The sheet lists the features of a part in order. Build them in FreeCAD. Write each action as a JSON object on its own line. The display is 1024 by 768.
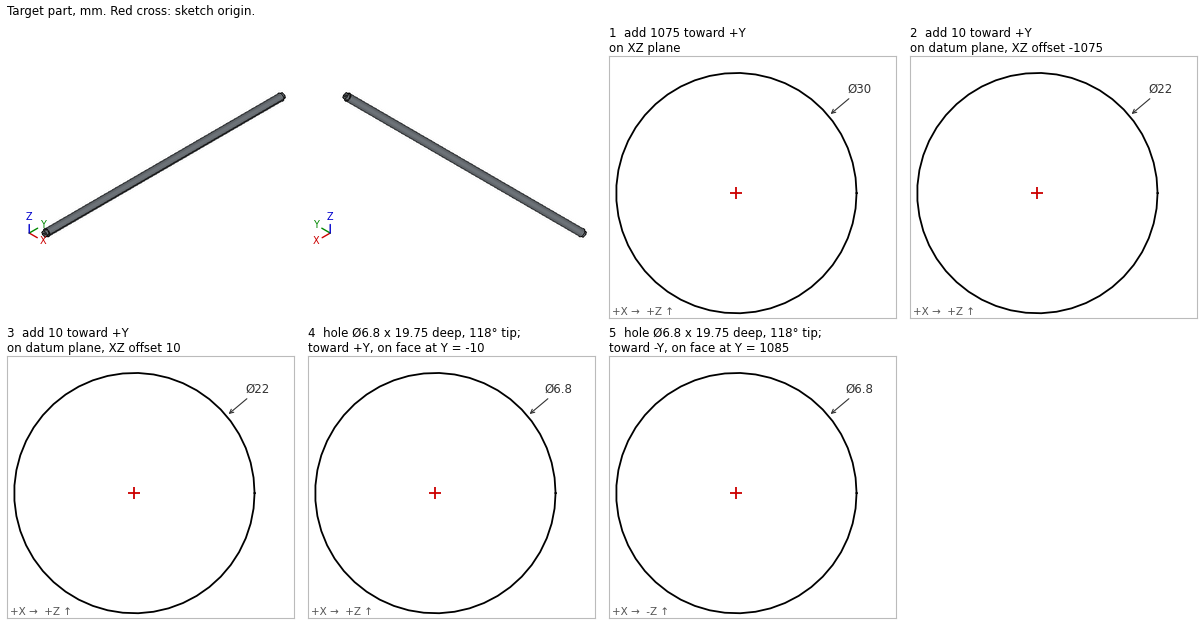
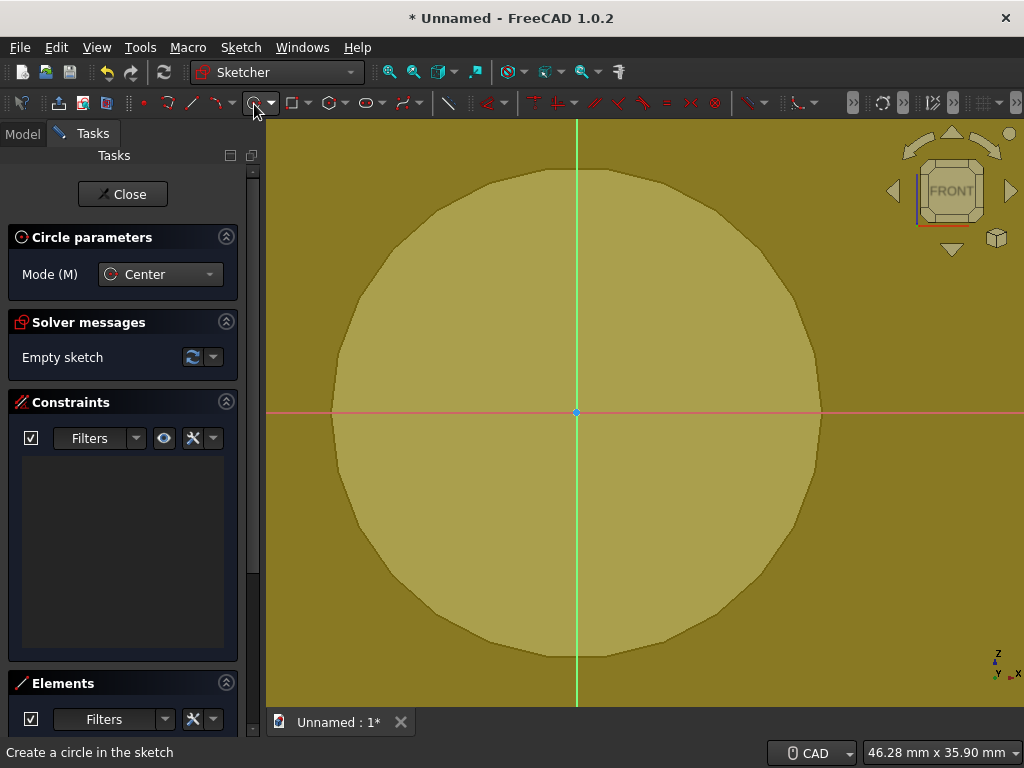
{"action": "left_click", "coordinate": [577, 413]}
{"action": "mouse_move", "coordinate": [704, 285]}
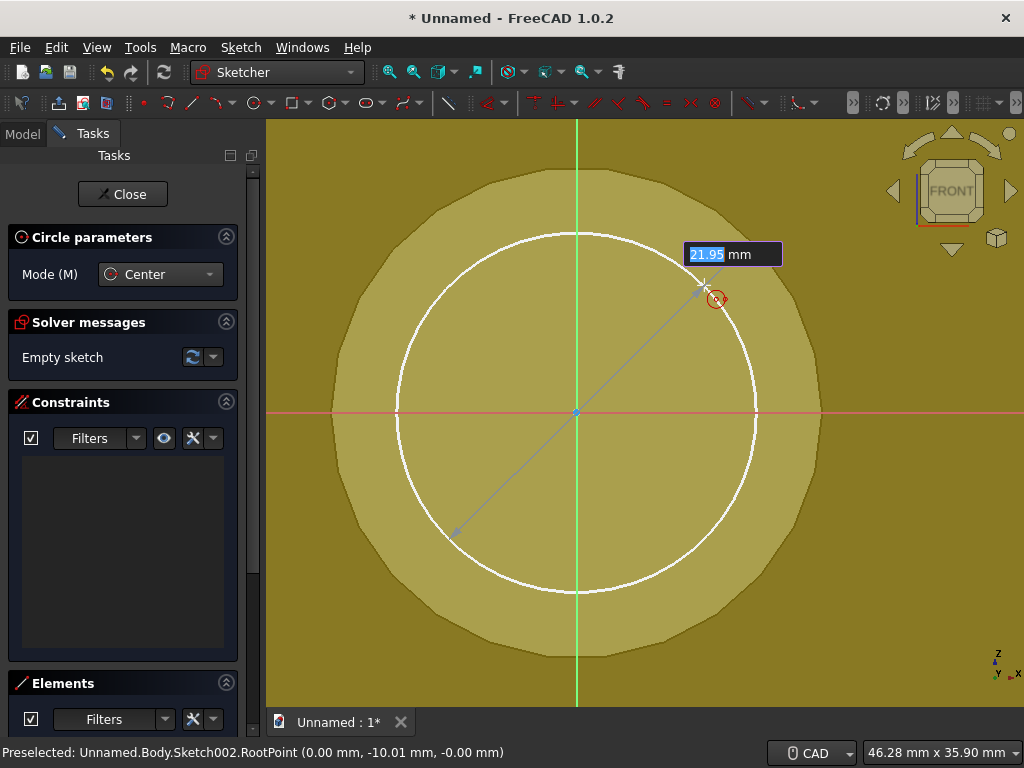
{"action": "type", "text": "22"}
{"action": "key", "text": "Return"}
{"action": "key", "text": "Escape"}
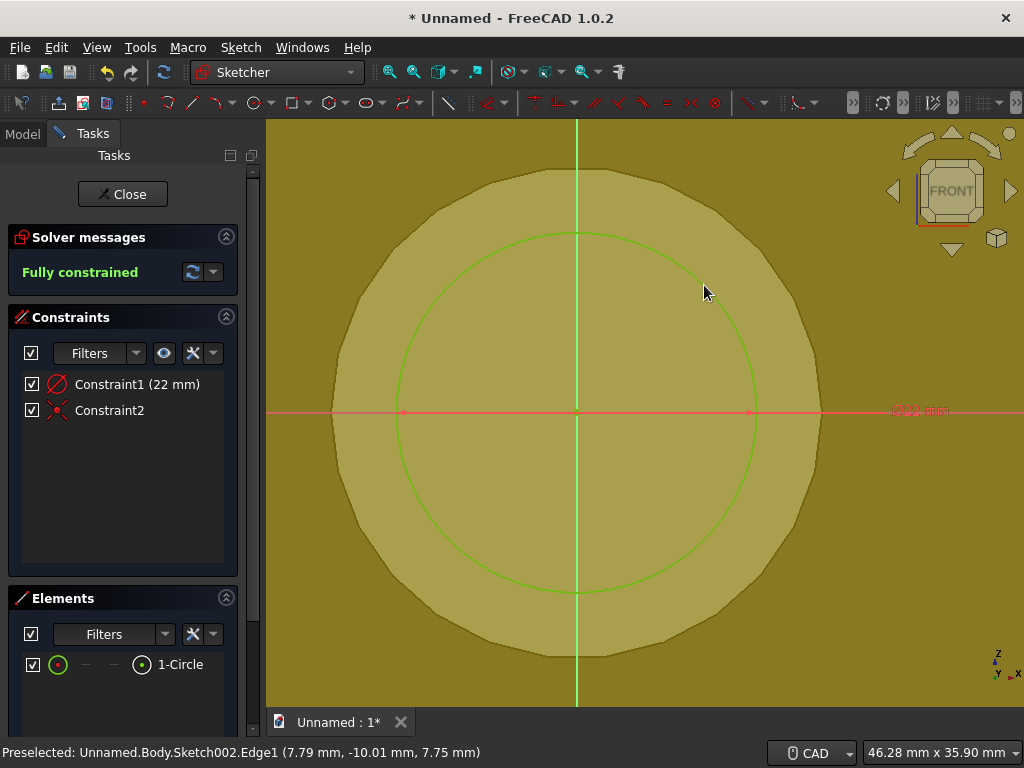
{"action": "left_click", "coordinate": [123, 194]}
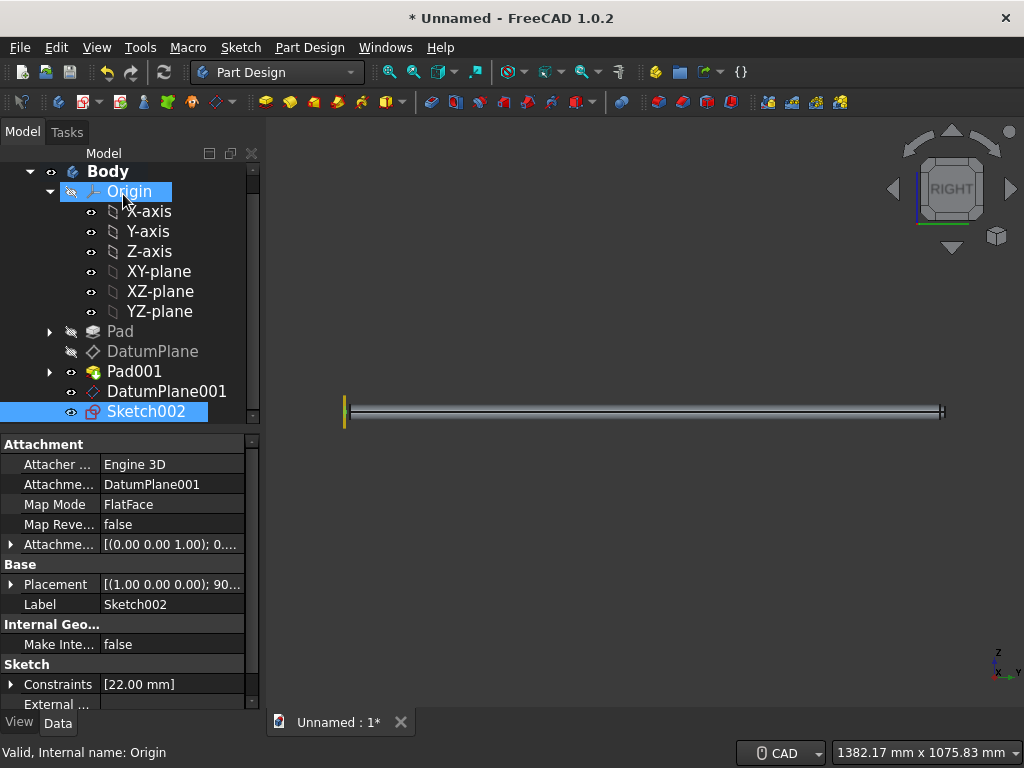
{"action": "left_click", "coordinate": [266, 102]}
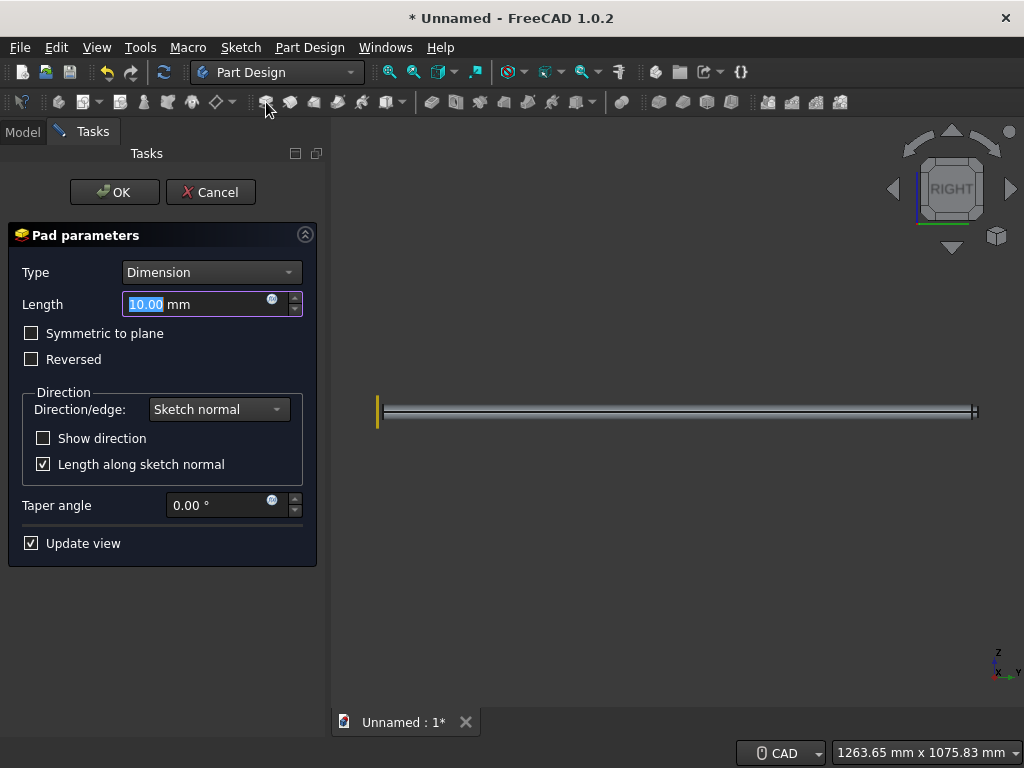
{"action": "type", "text": "10"}
{"action": "key", "text": "Tab"}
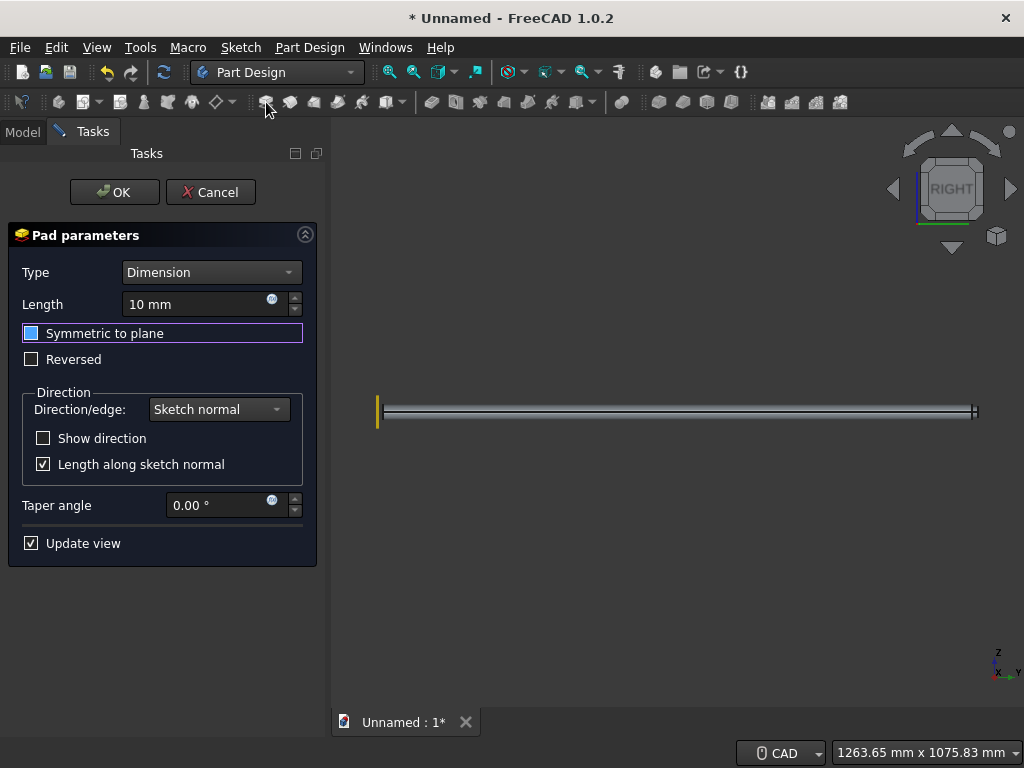
{"action": "left_click", "coordinate": [30, 359]}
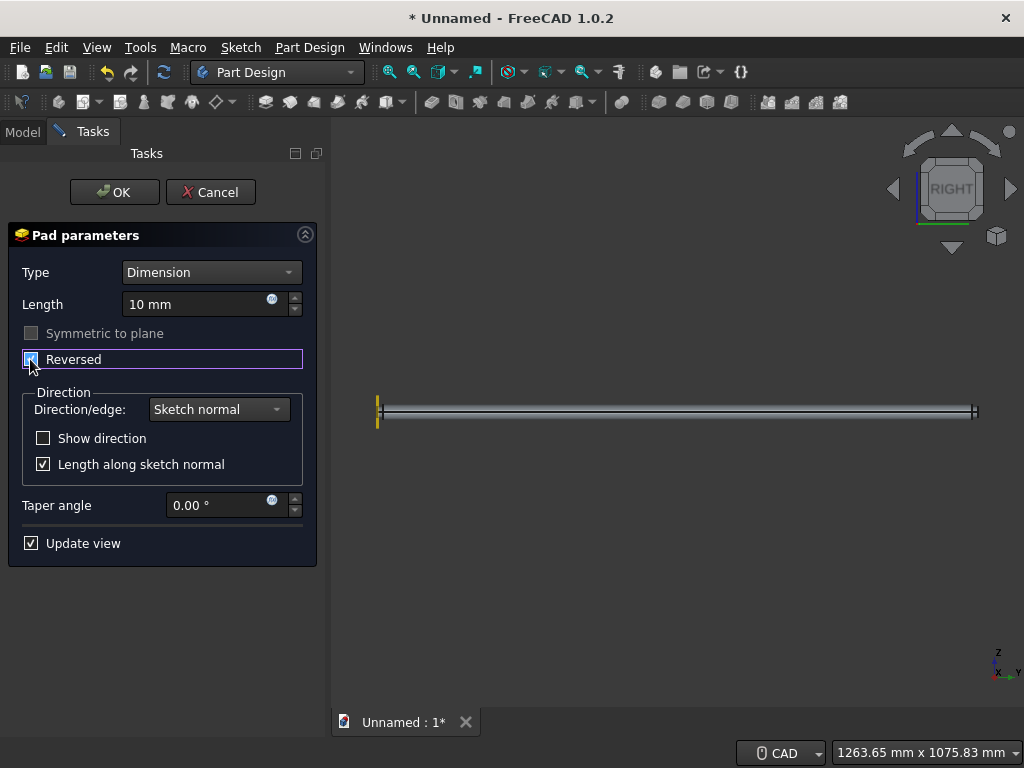
{"action": "left_click", "coordinate": [115, 192]}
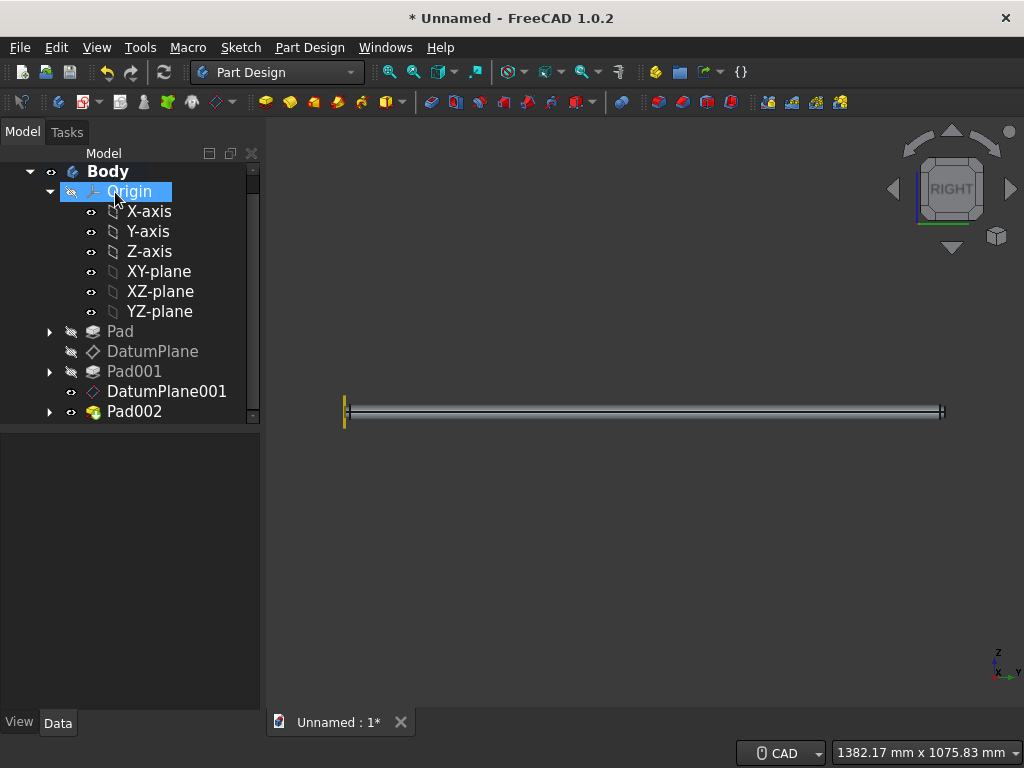
{"action": "left_click", "coordinate": [116, 392]}
{"action": "key", "text": "space"}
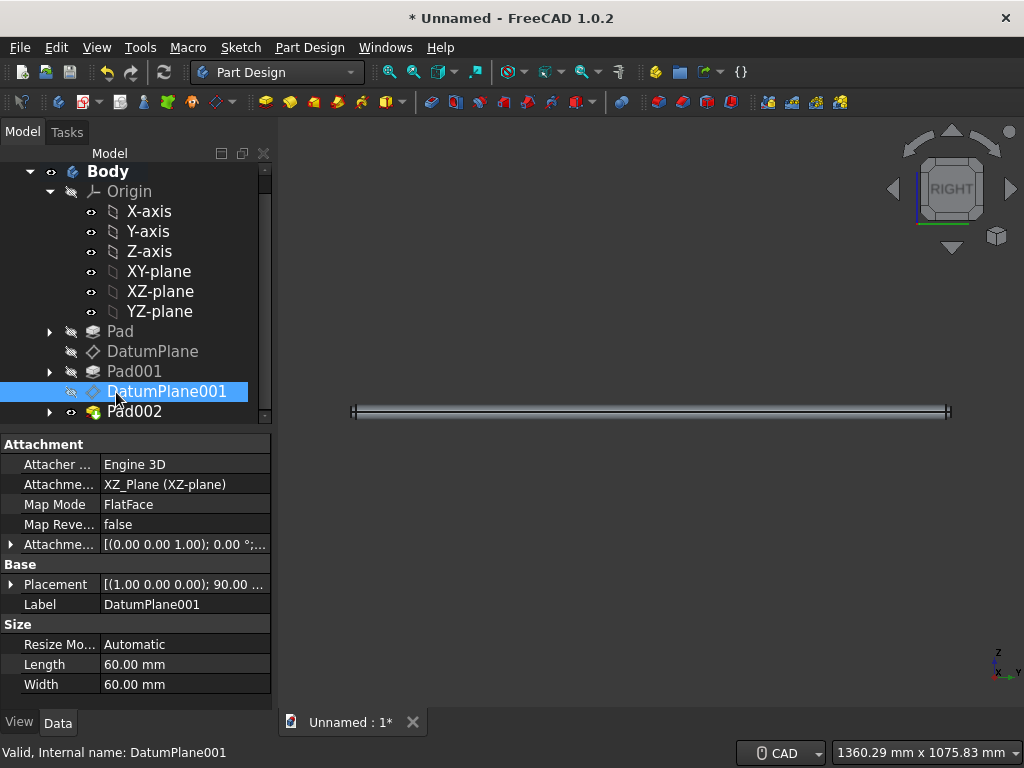
{"action": "key", "text": "0"}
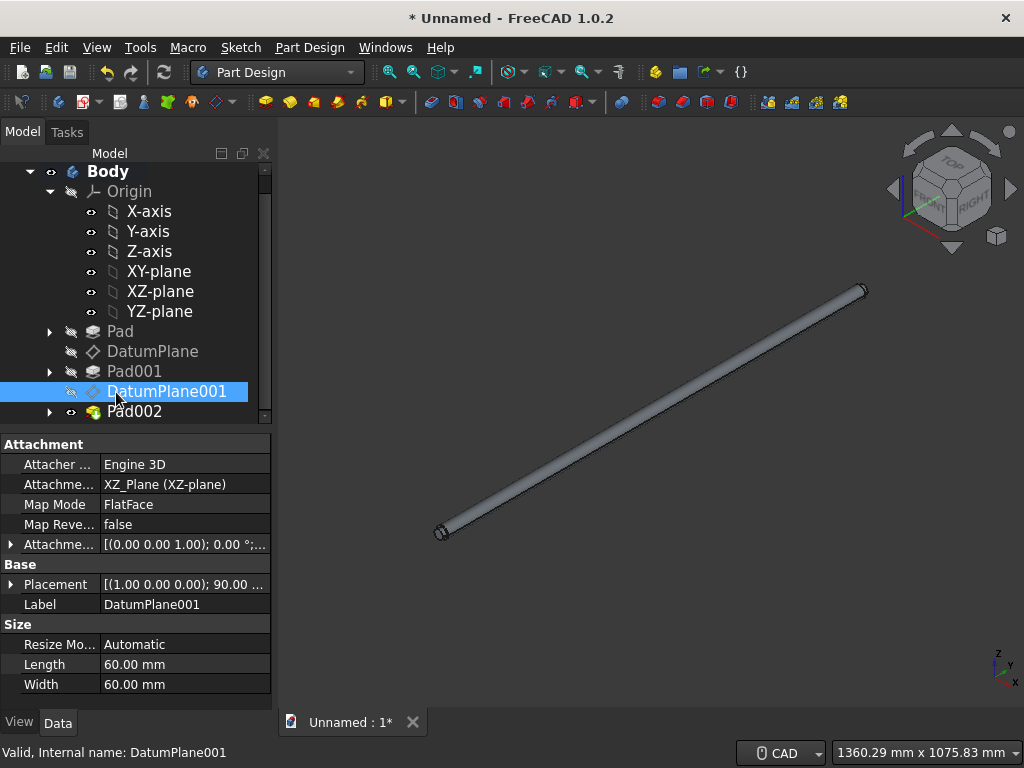
{"action": "scroll", "coordinate": [439, 534], "scroll_direction": "up", "scroll_amount": 4}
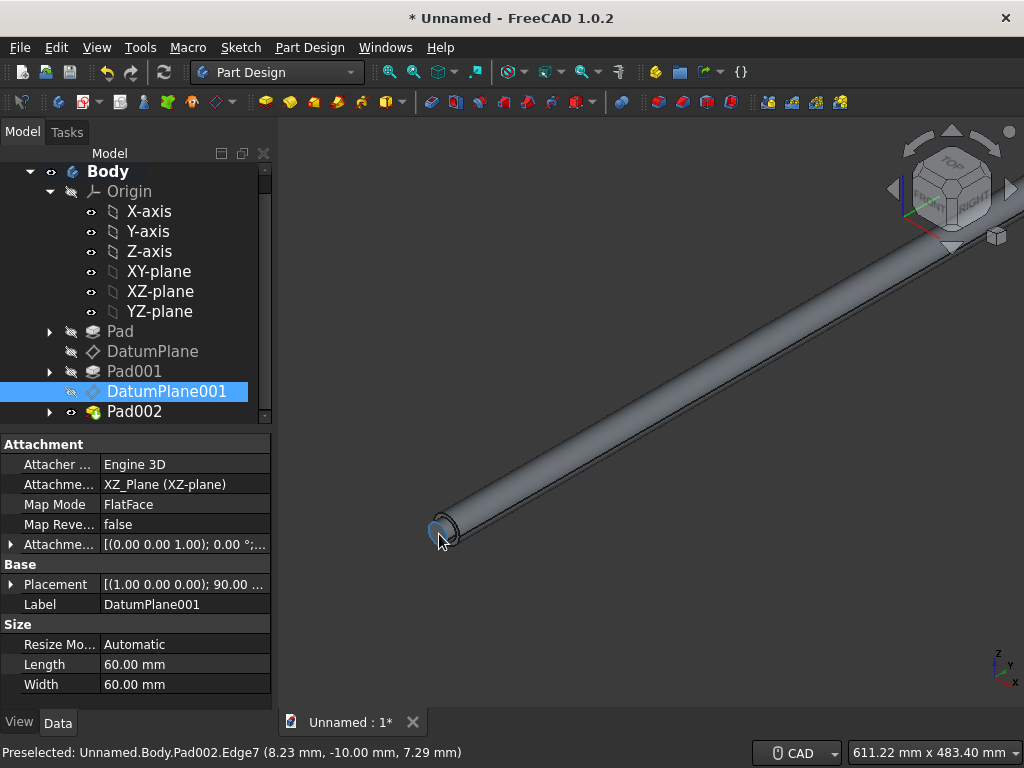
{"action": "left_click", "coordinate": [438, 537]}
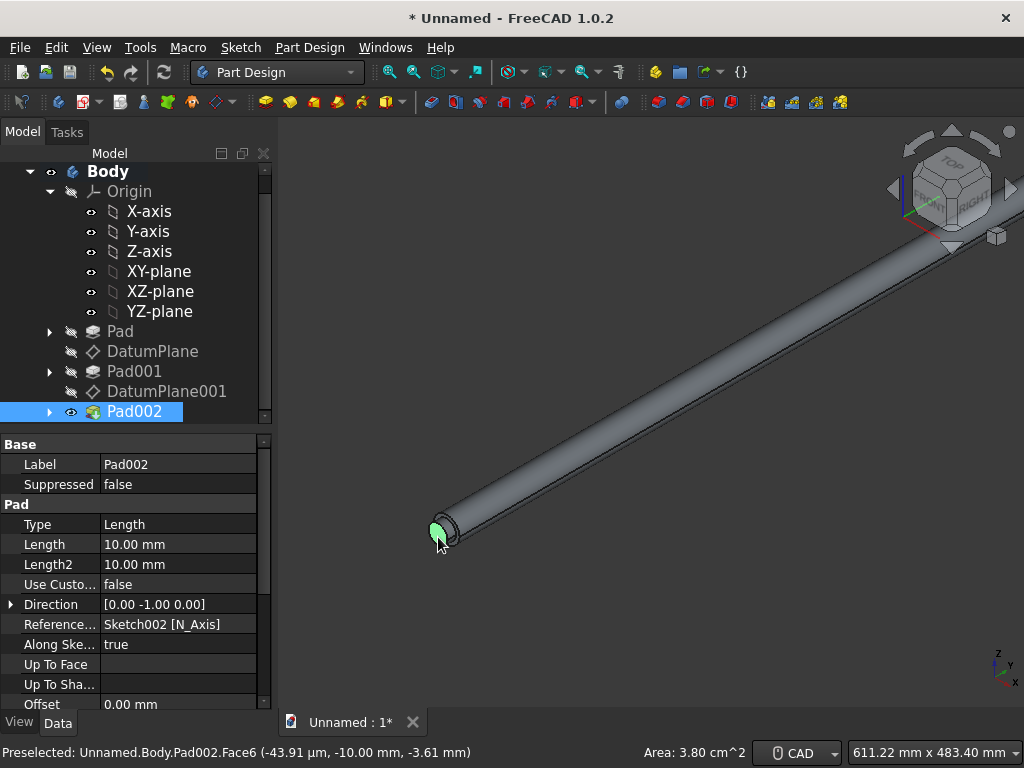
{"action": "left_click", "coordinate": [84, 102]}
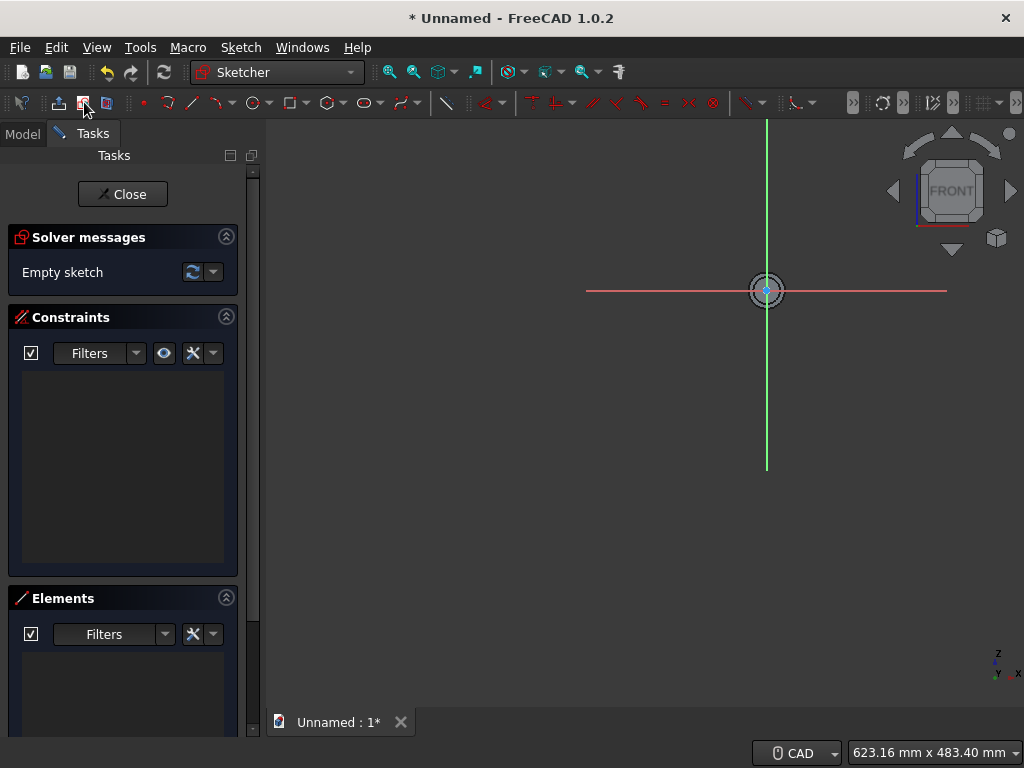
{"action": "scroll", "coordinate": [777, 284], "scroll_direction": "up", "scroll_amount": 15}